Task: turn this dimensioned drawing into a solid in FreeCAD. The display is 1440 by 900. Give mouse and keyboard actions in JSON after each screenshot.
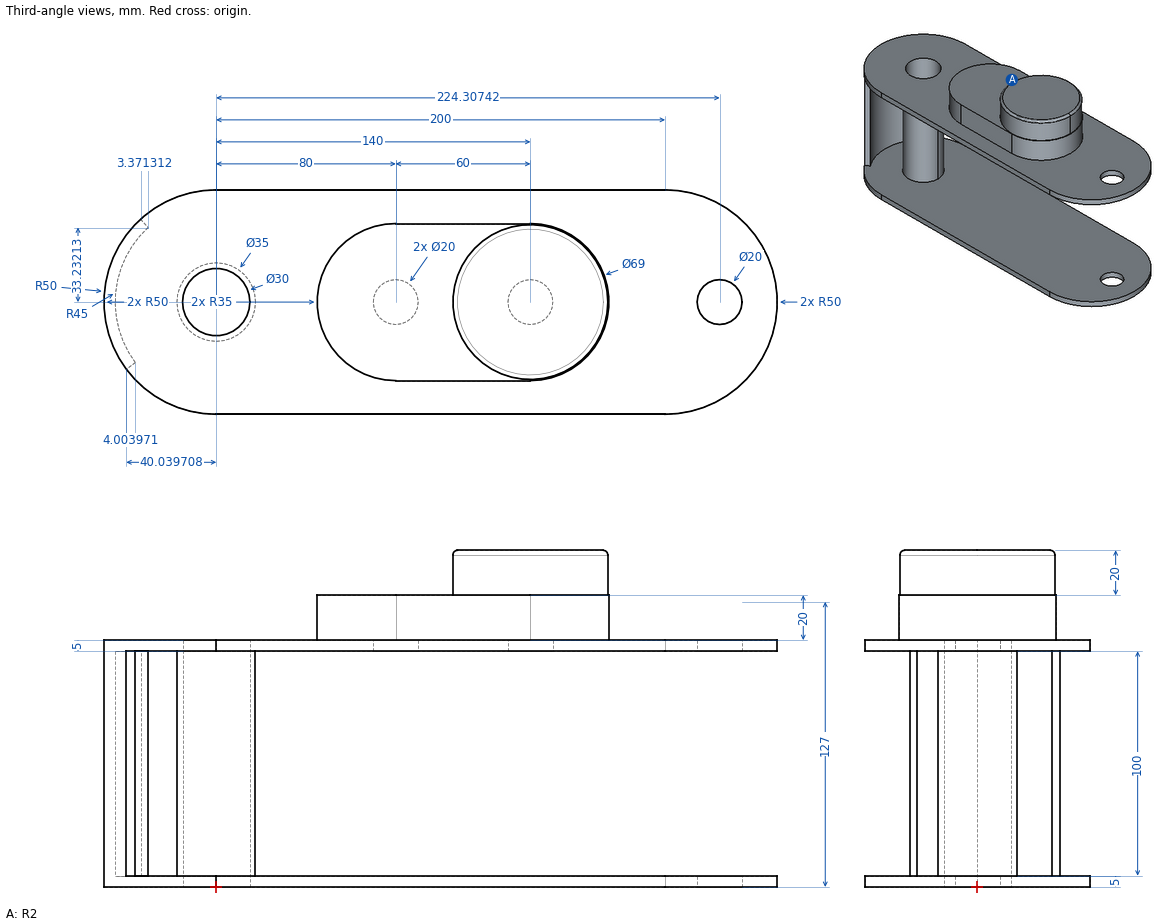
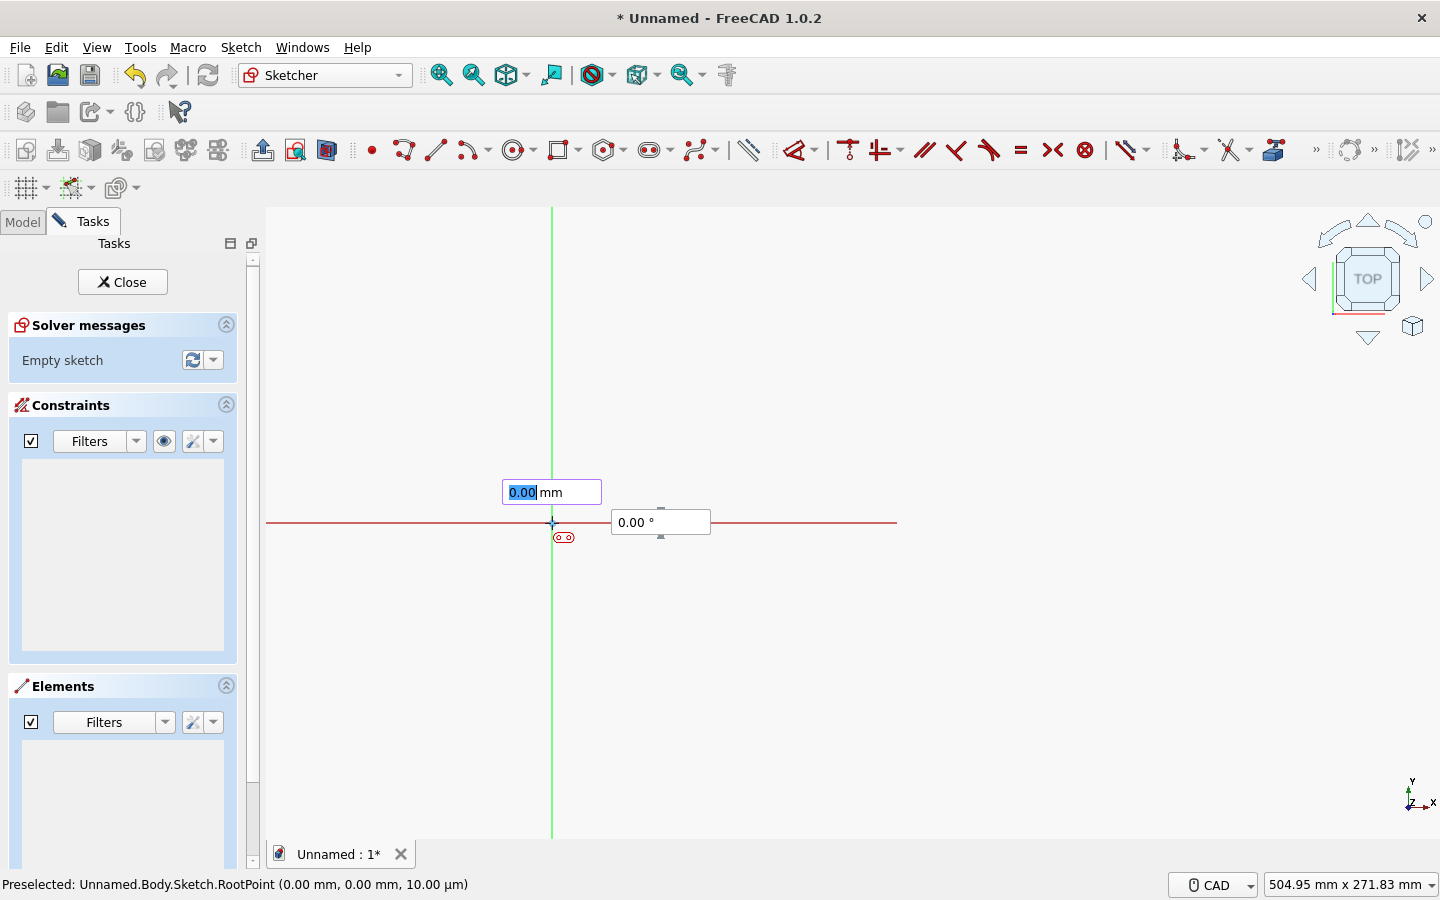
{"action": "left_click", "coordinate": [1017, 514]}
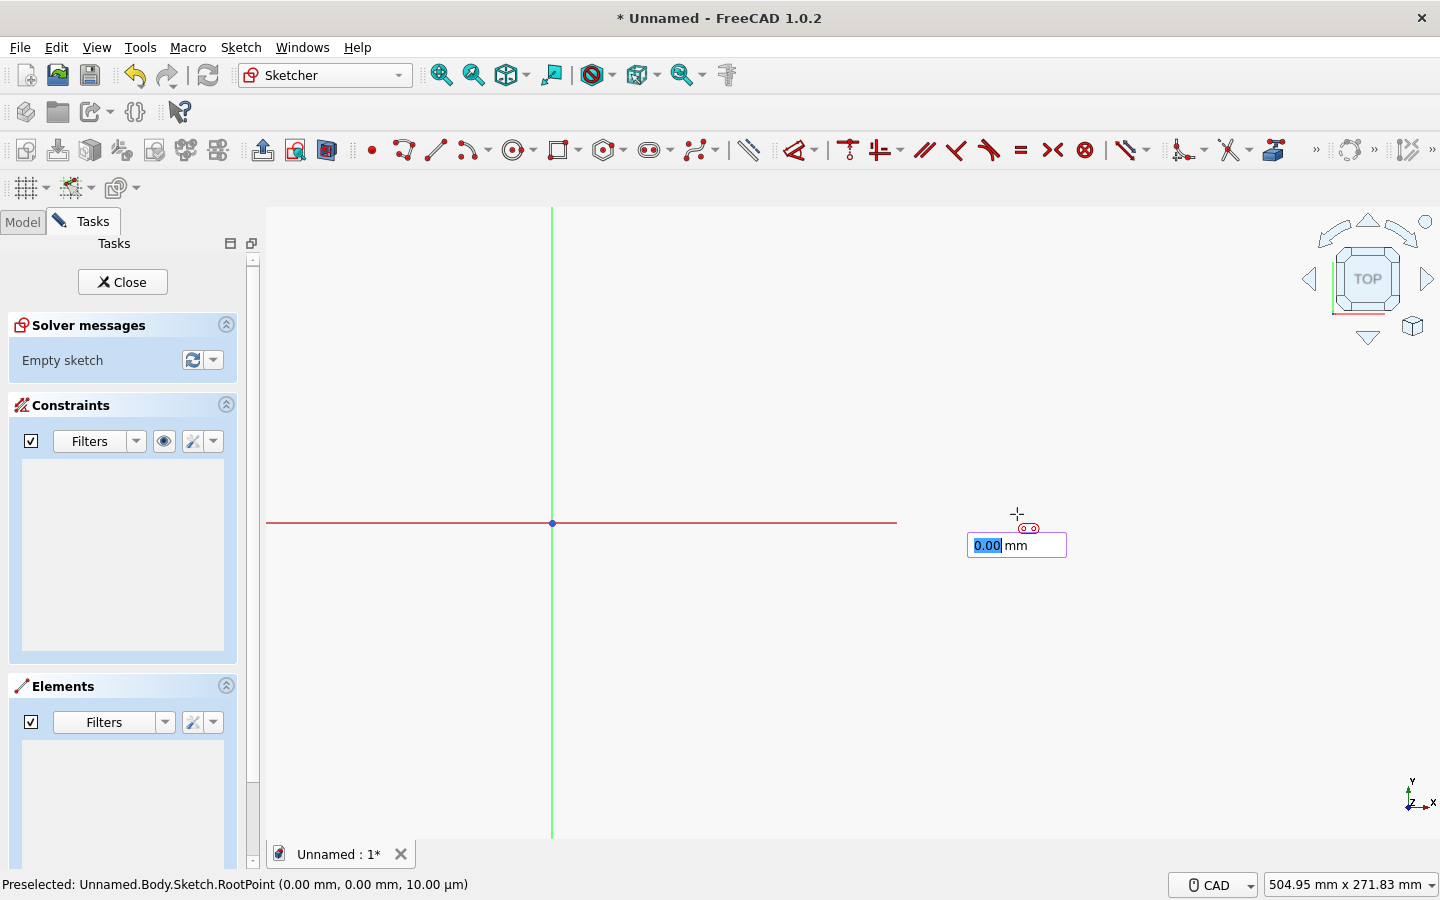
{"action": "left_click", "coordinate": [785, 407]}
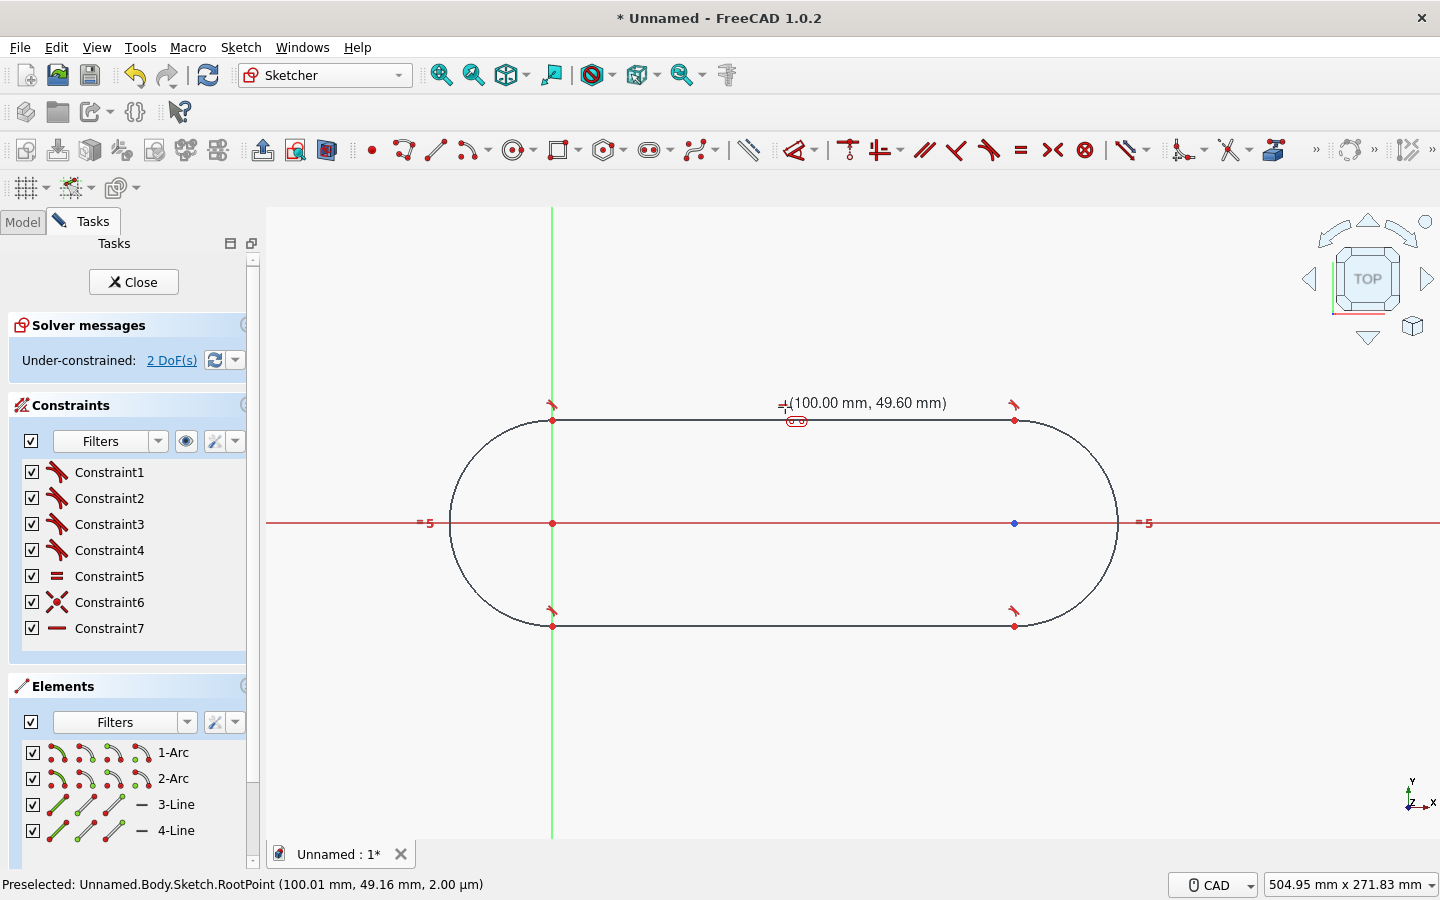
{"action": "left_click", "coordinate": [514, 150]}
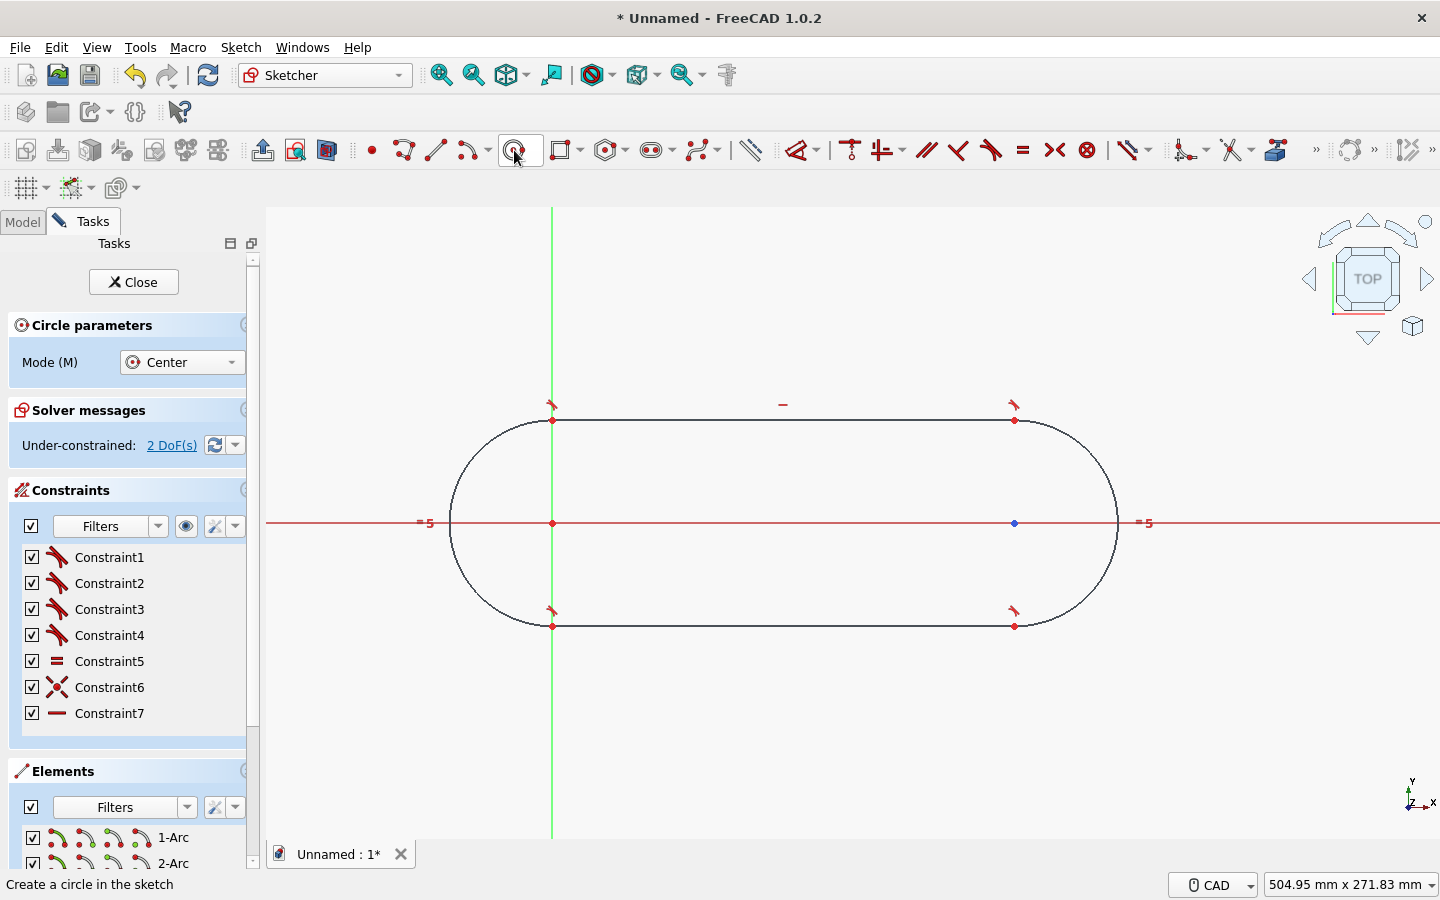
{"action": "left_click", "coordinate": [552, 523]}
{"action": "left_click", "coordinate": [577, 499]}
{"action": "key", "text": "Escape"}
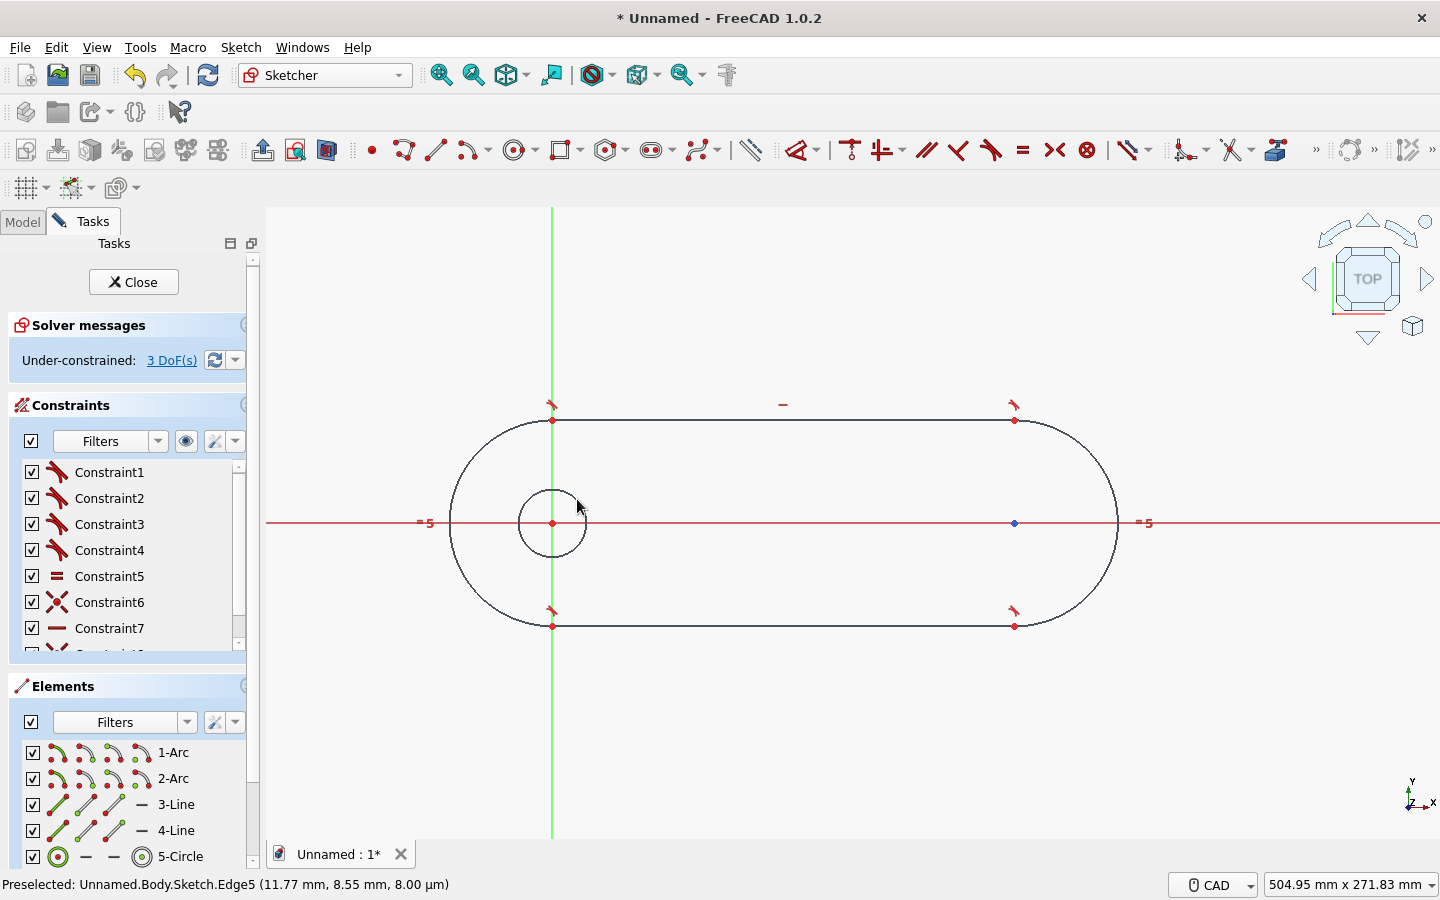
{"action": "left_click", "coordinate": [796, 150]}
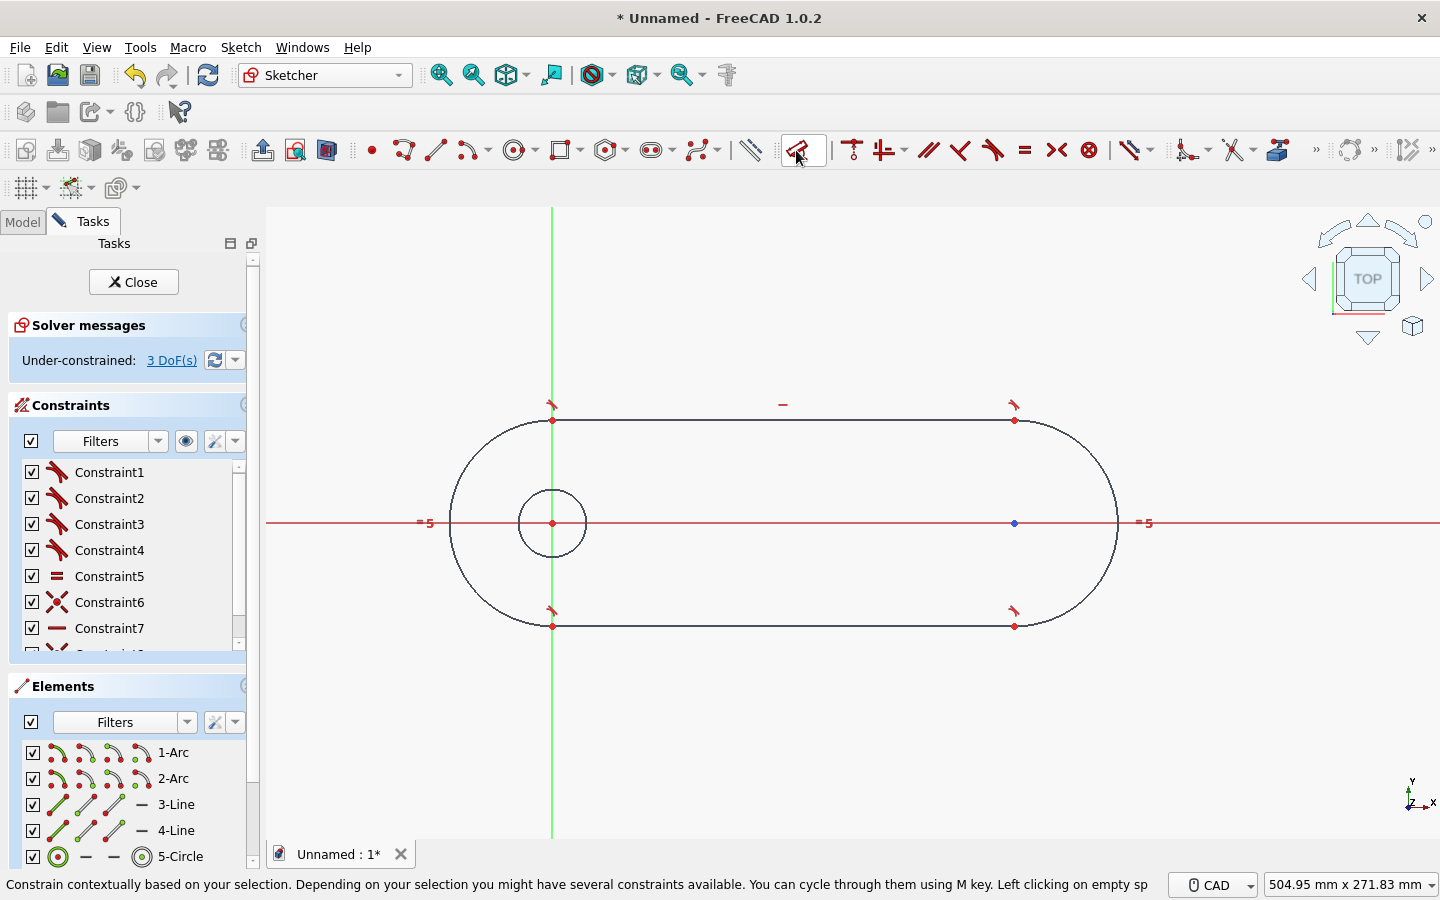
{"action": "left_click", "coordinate": [469, 463]}
{"action": "left_click", "coordinate": [443, 444]}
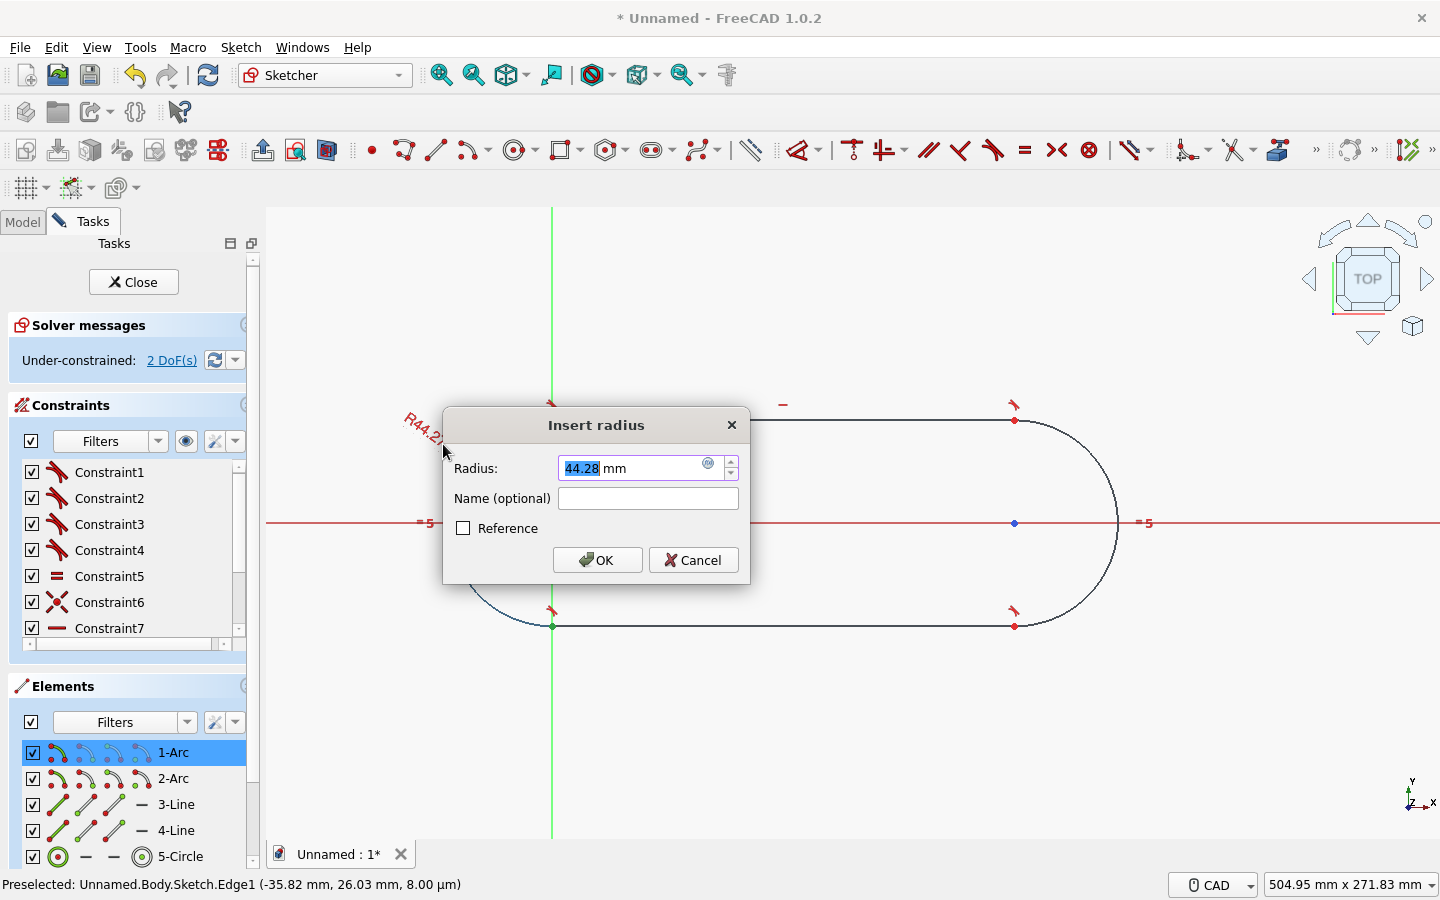
{"action": "type", "text": "50"}
{"action": "key", "text": "Return"}